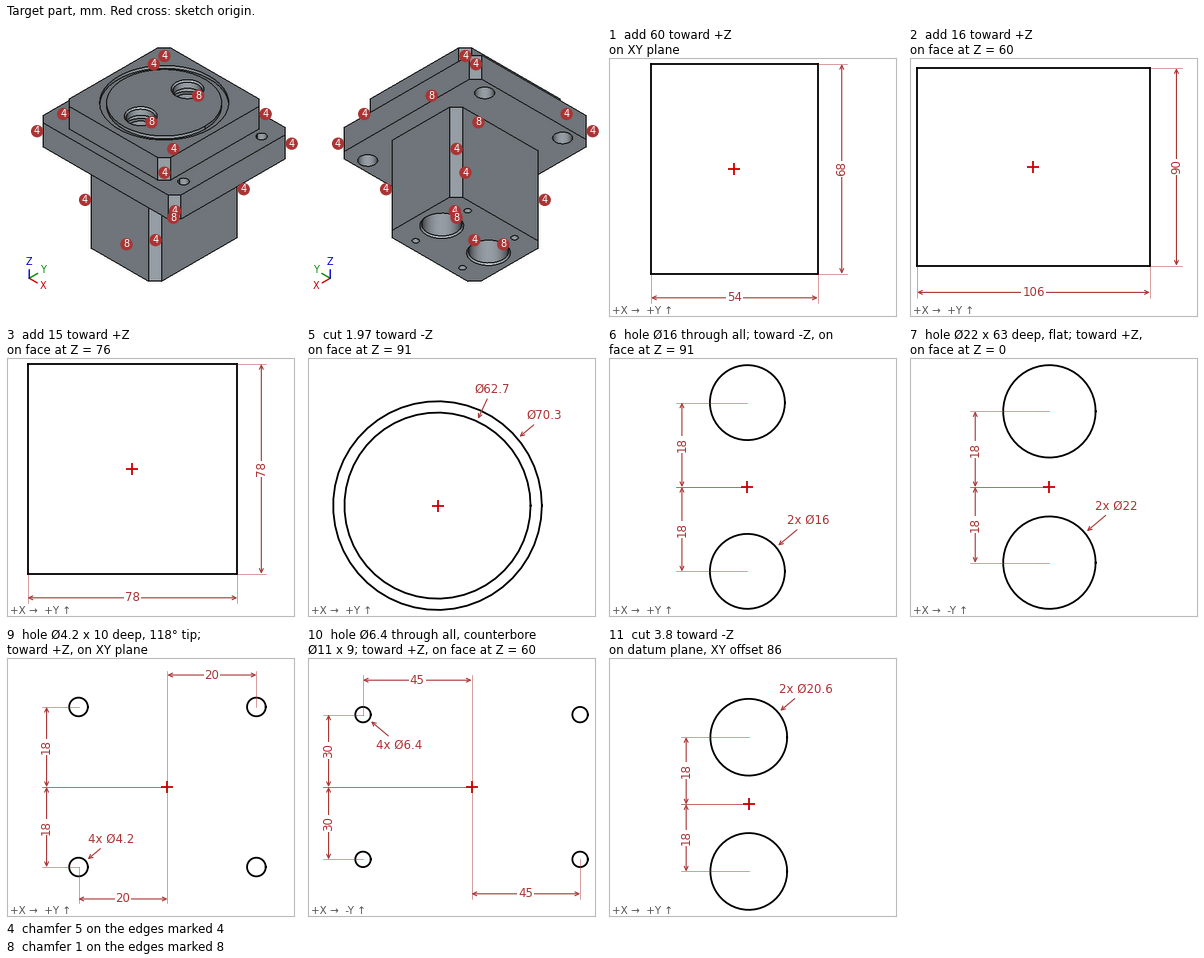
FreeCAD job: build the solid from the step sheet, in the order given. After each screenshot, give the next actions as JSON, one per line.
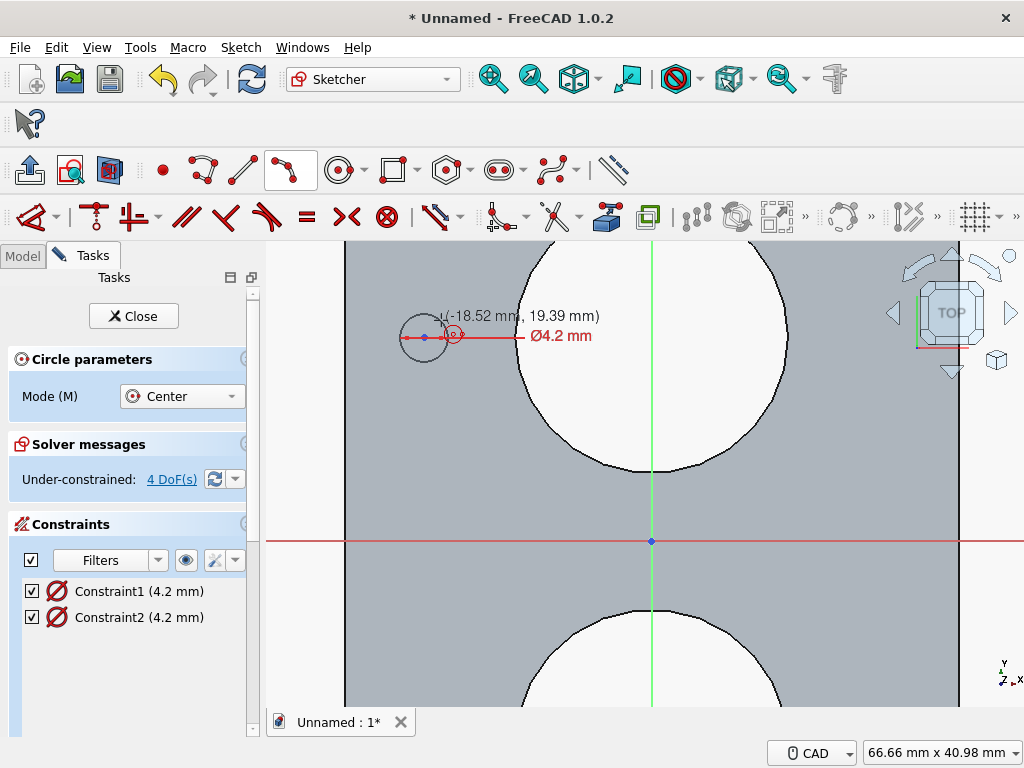
{"action": "scroll", "coordinate": [424, 337], "scroll_direction": "down", "scroll_amount": 2}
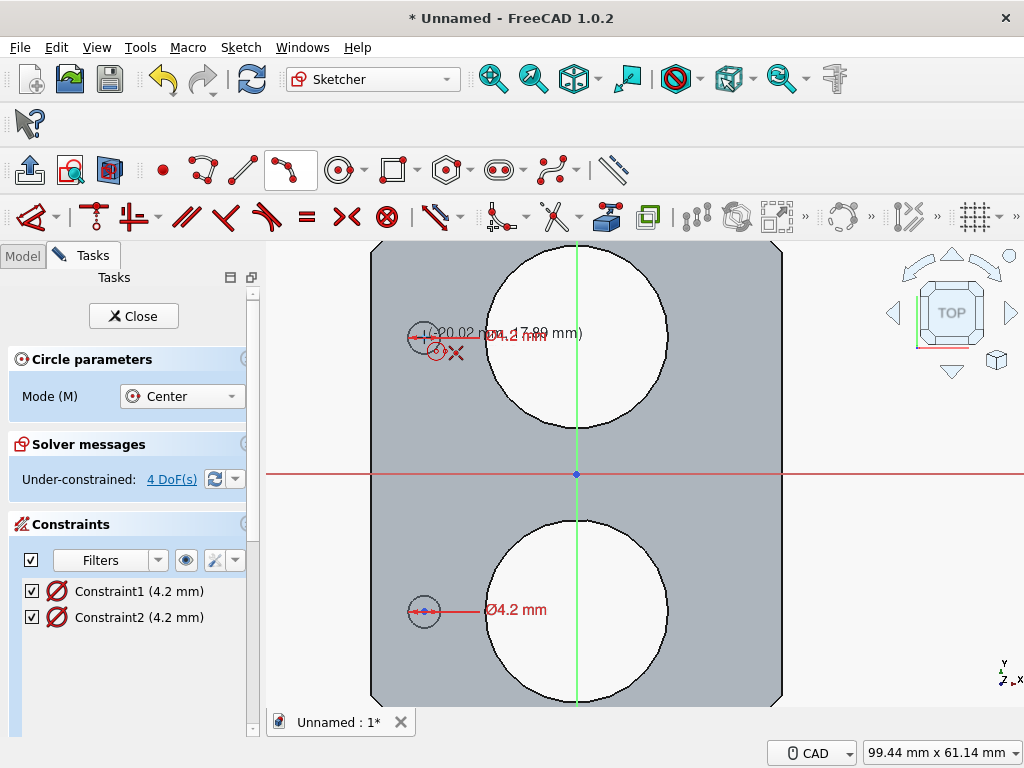
{"action": "scroll", "coordinate": [729, 337], "scroll_direction": "up", "scroll_amount": 2}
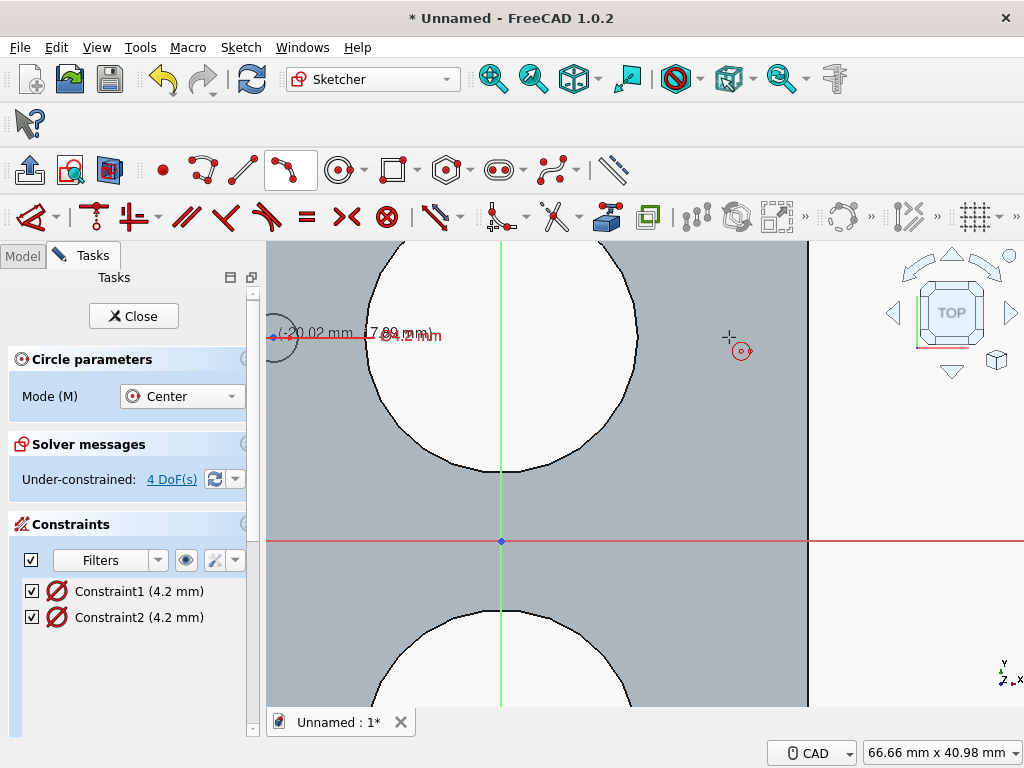
{"action": "left_click", "coordinate": [729, 337]}
{"action": "mouse_move", "coordinate": [746, 320]}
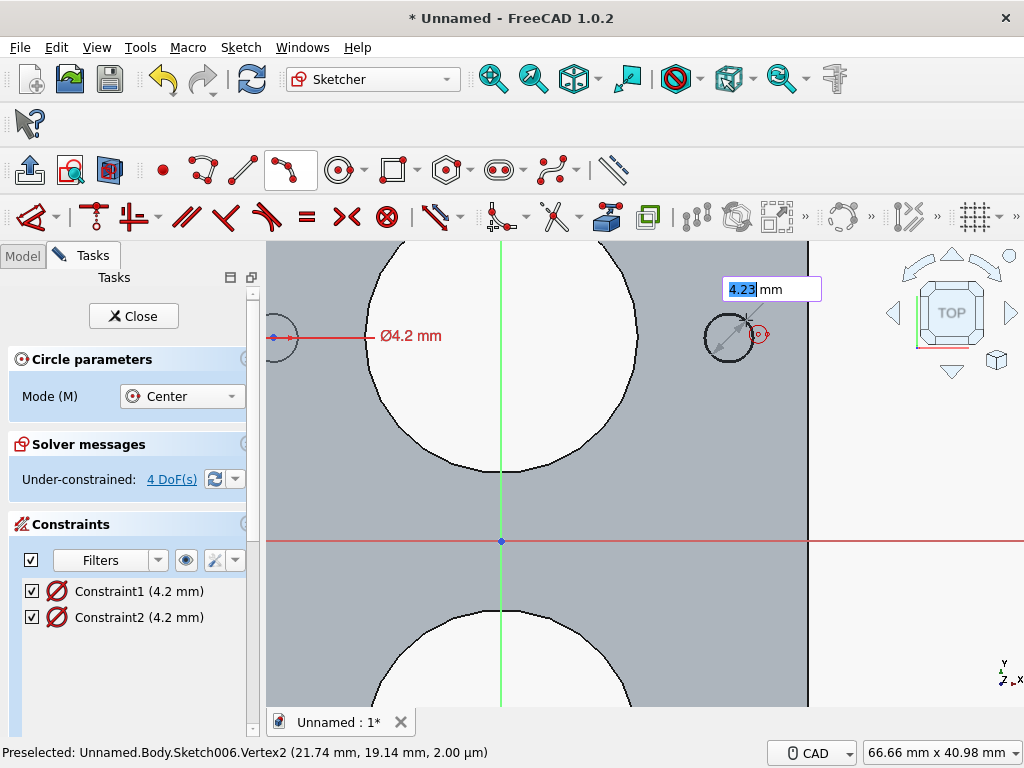
{"action": "type", "text": "4.2"}
{"action": "key", "text": "Return"}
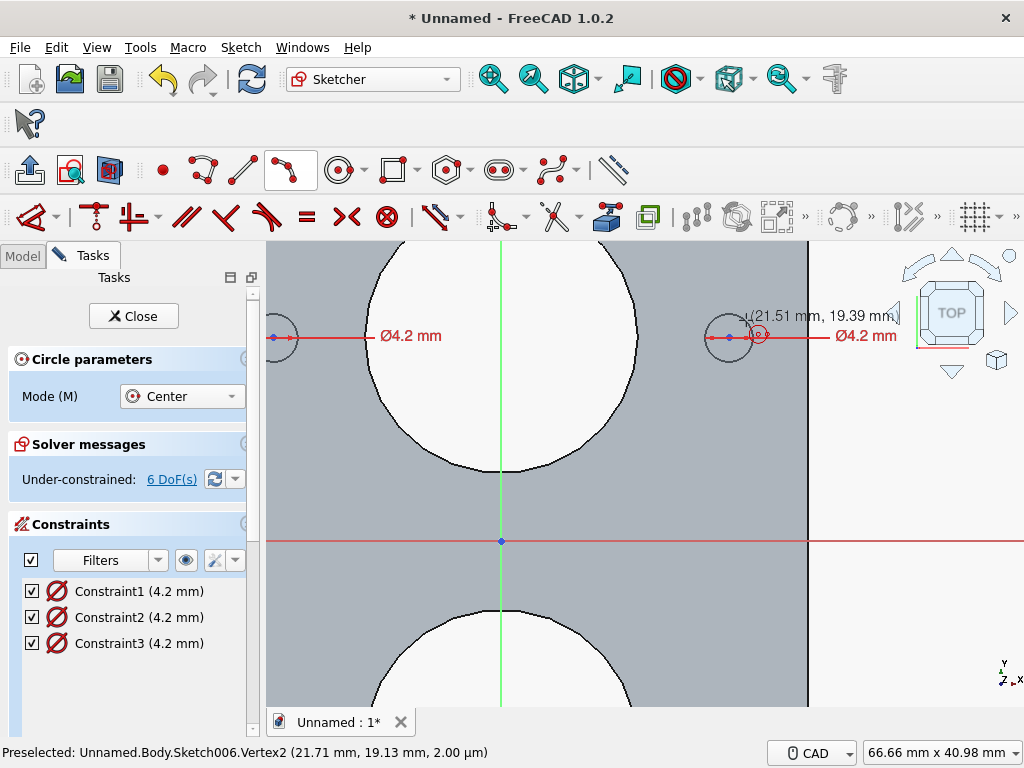
{"action": "scroll", "coordinate": [729, 337], "scroll_direction": "down", "scroll_amount": 2}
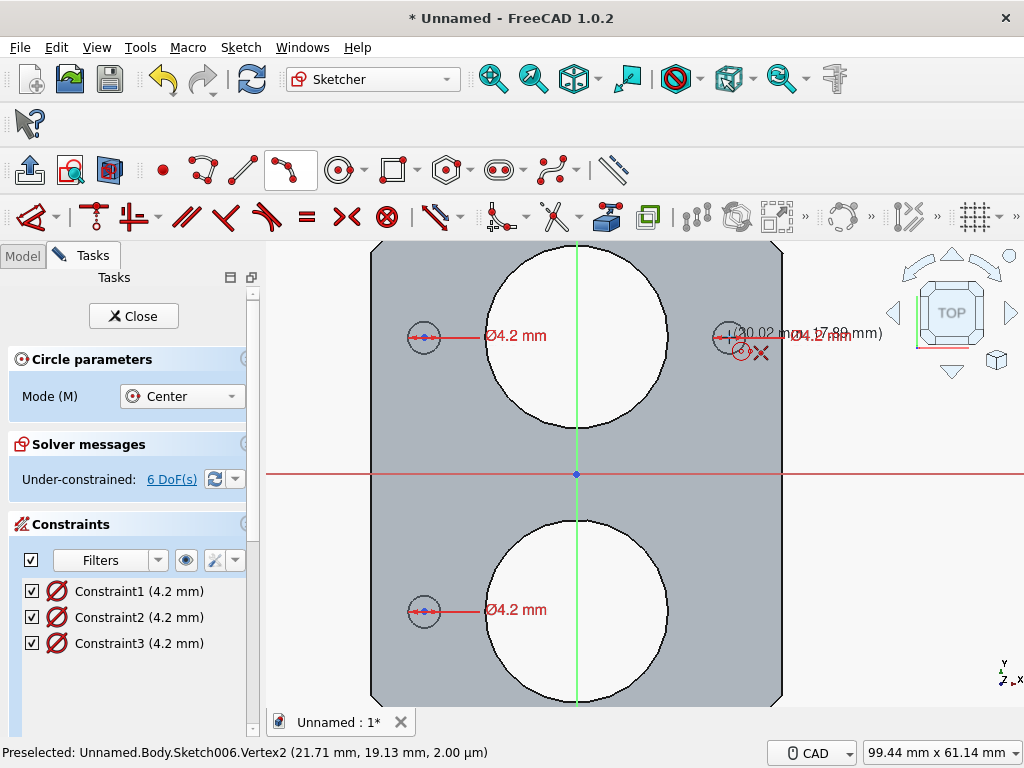
{"action": "scroll", "coordinate": [729, 611], "scroll_direction": "up", "scroll_amount": 2}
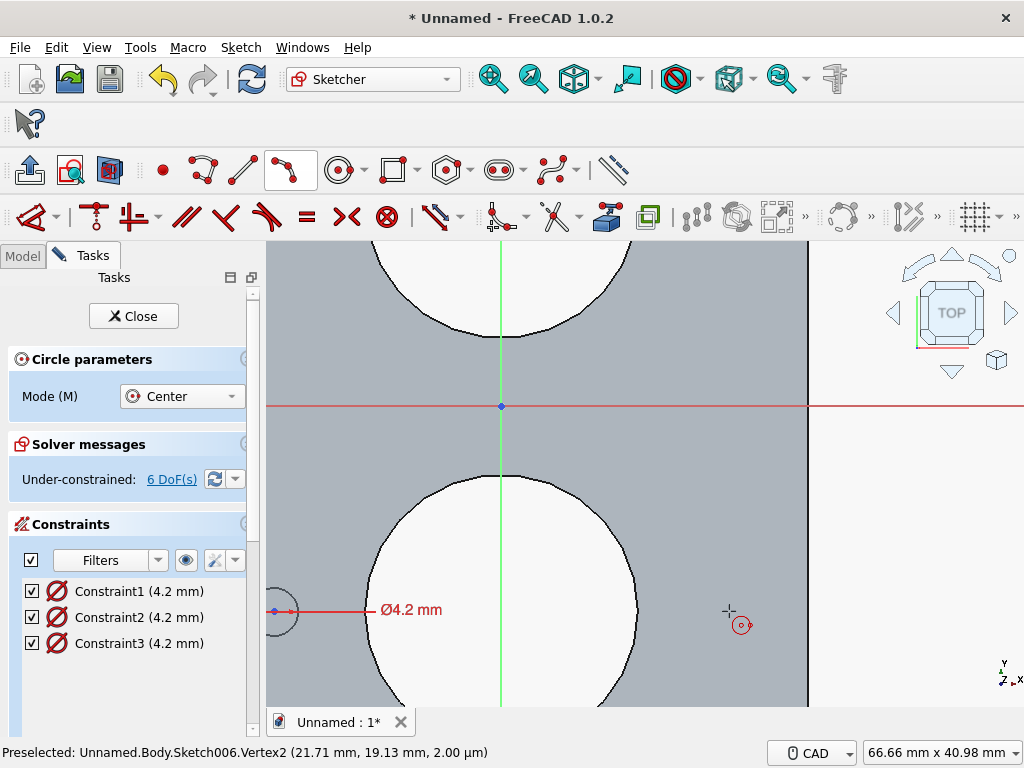
{"action": "left_click", "coordinate": [729, 611]}
{"action": "mouse_move", "coordinate": [746, 594]}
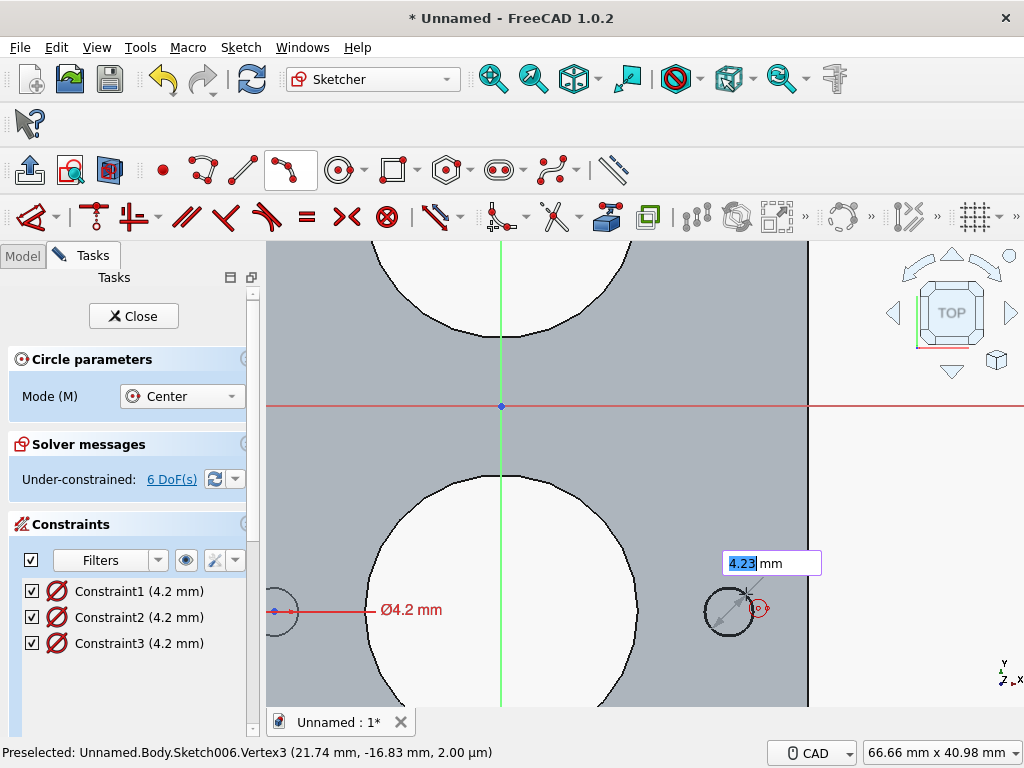
{"action": "type", "text": "4.2"}
{"action": "key", "text": "Return"}
{"action": "key", "text": "Escape"}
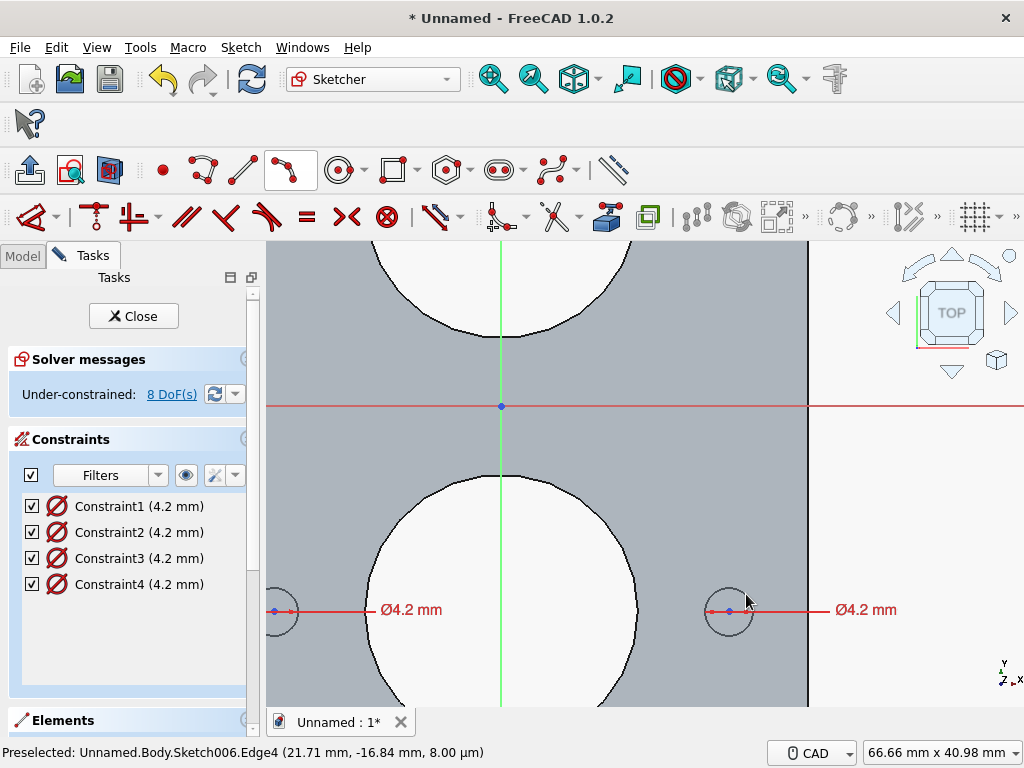
{"action": "scroll", "coordinate": [729, 611], "scroll_direction": "down", "scroll_amount": 2}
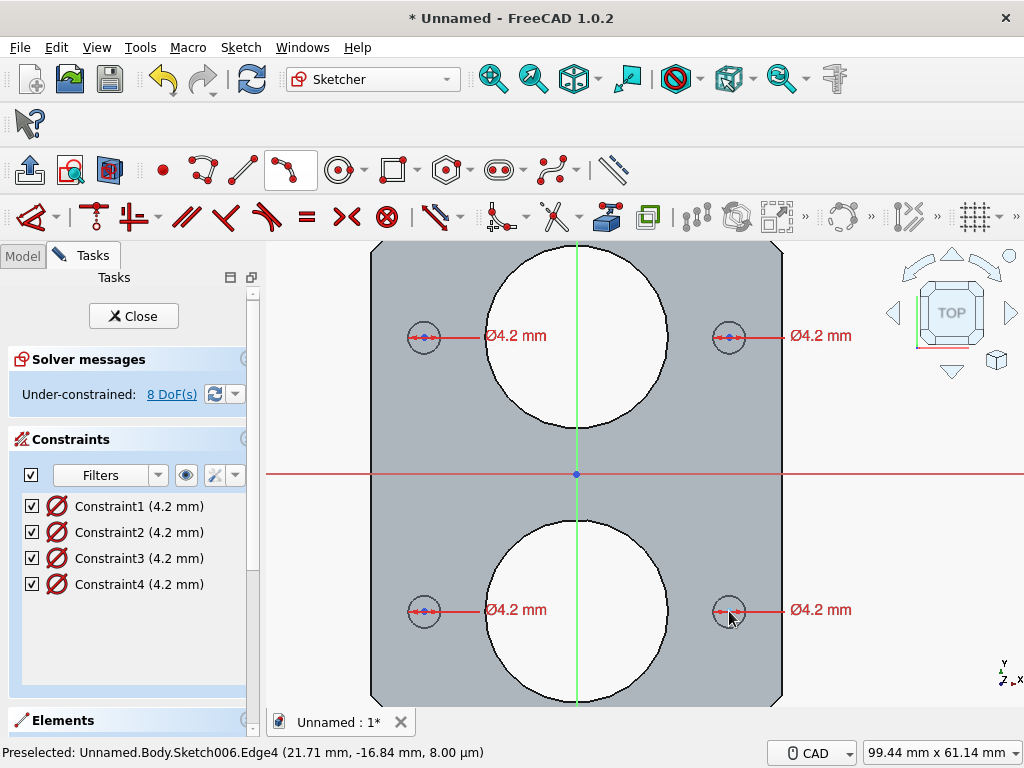
{"action": "left_click", "coordinate": [424, 612]}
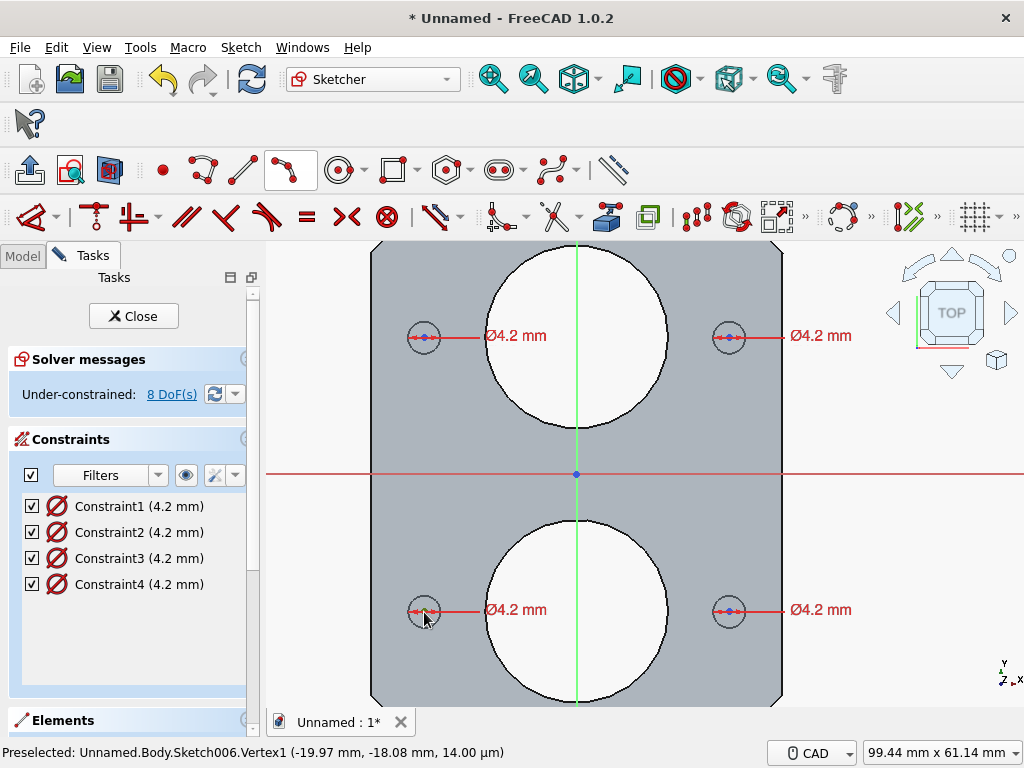
{"action": "left_click", "coordinate": [424, 338]}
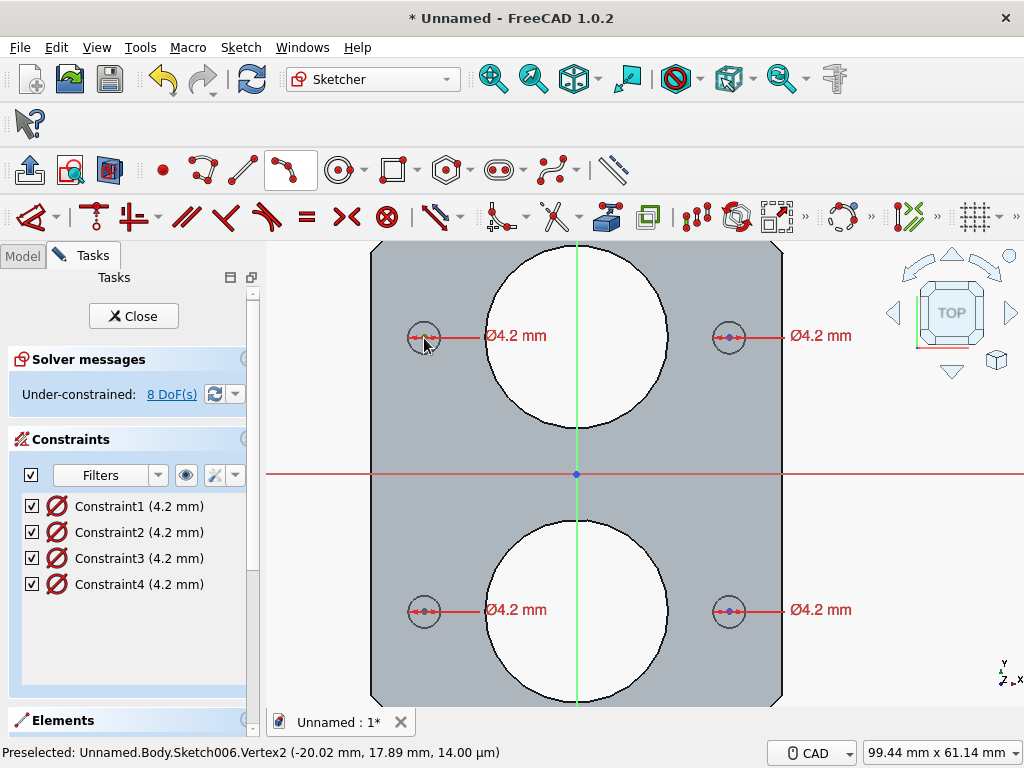
{"action": "key", "text": "v"}